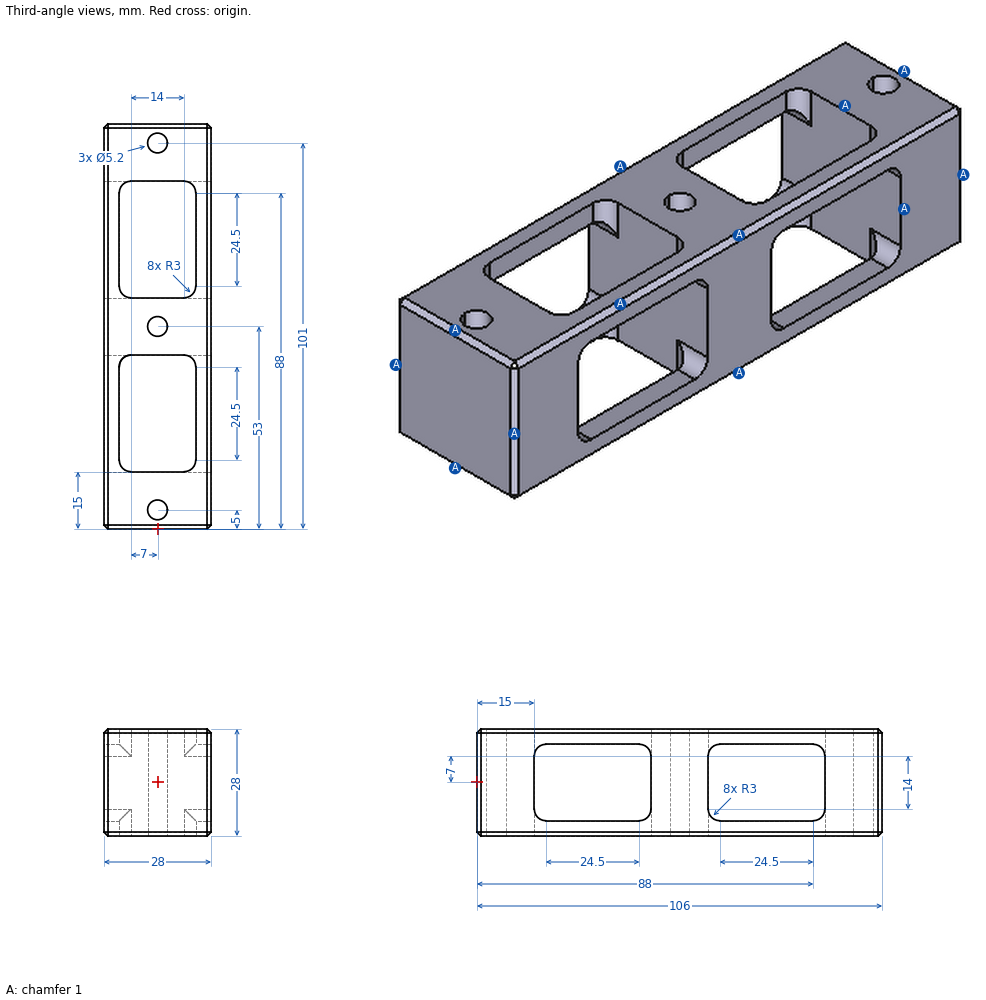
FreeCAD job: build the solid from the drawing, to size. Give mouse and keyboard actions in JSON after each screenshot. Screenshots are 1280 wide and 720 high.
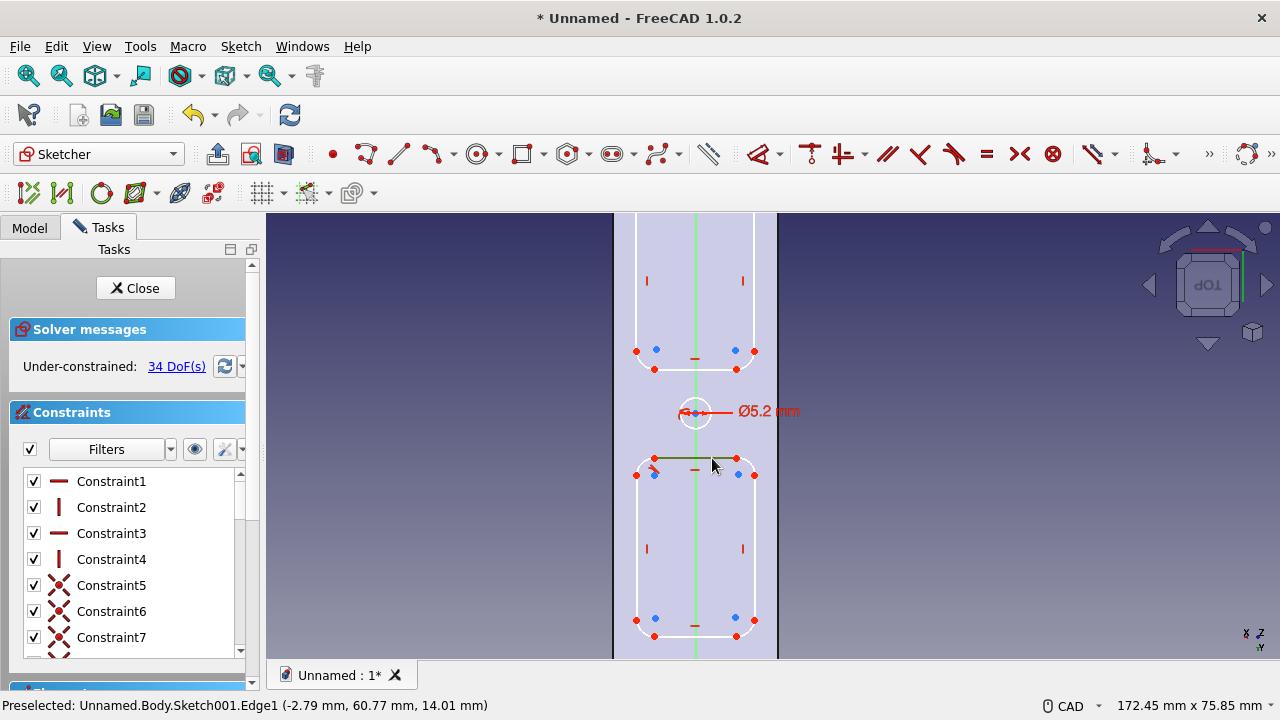
{"action": "left_click", "coordinate": [750, 463]}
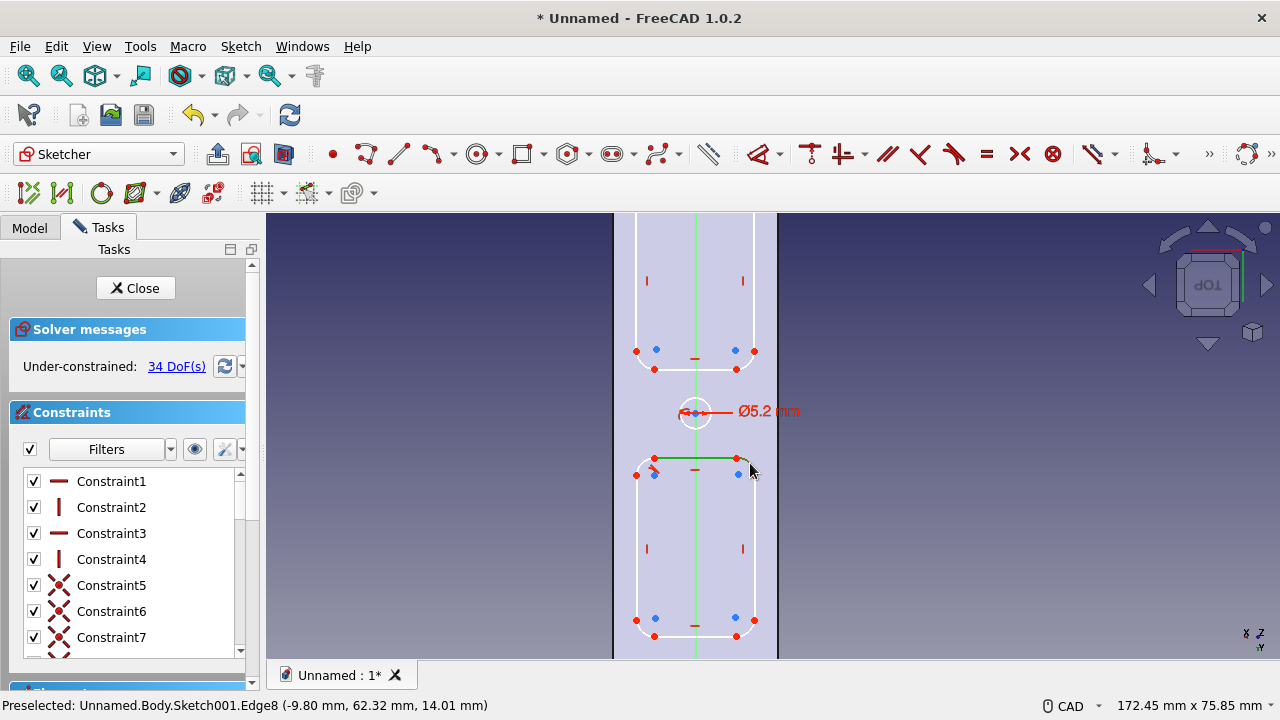
{"action": "left_click", "coordinate": [954, 154]}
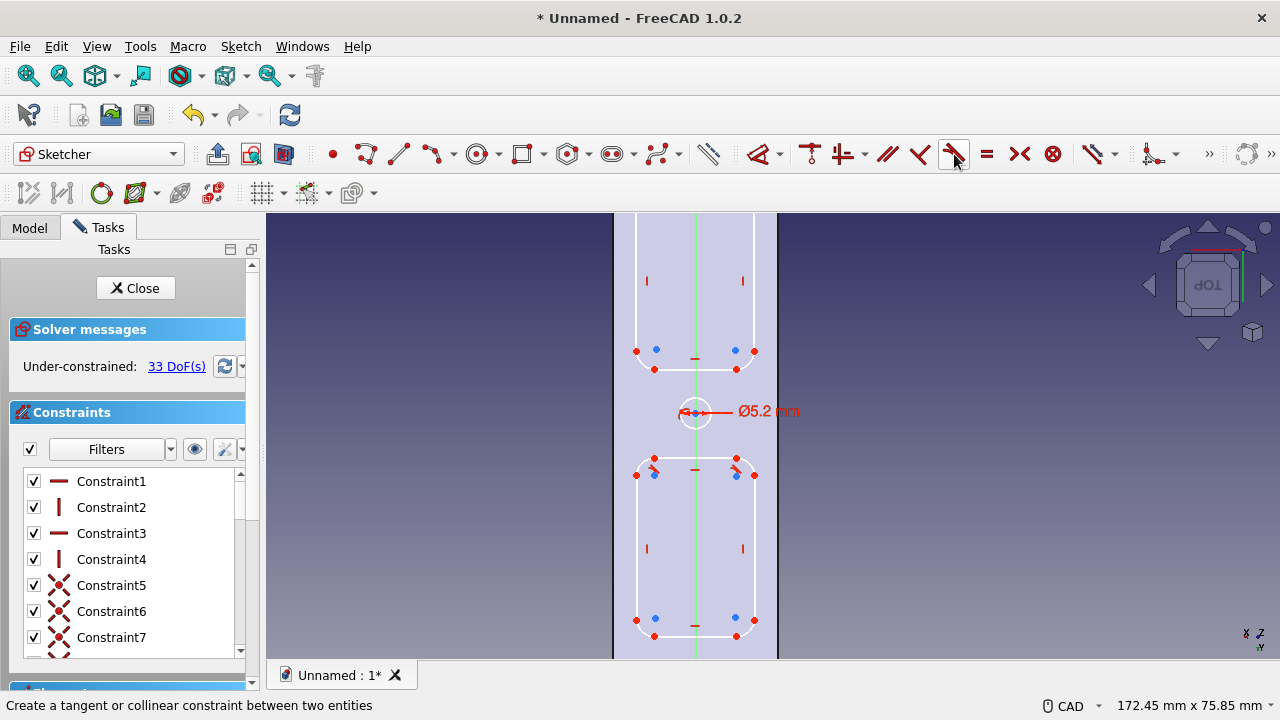
{"action": "left_click", "coordinate": [637, 519]}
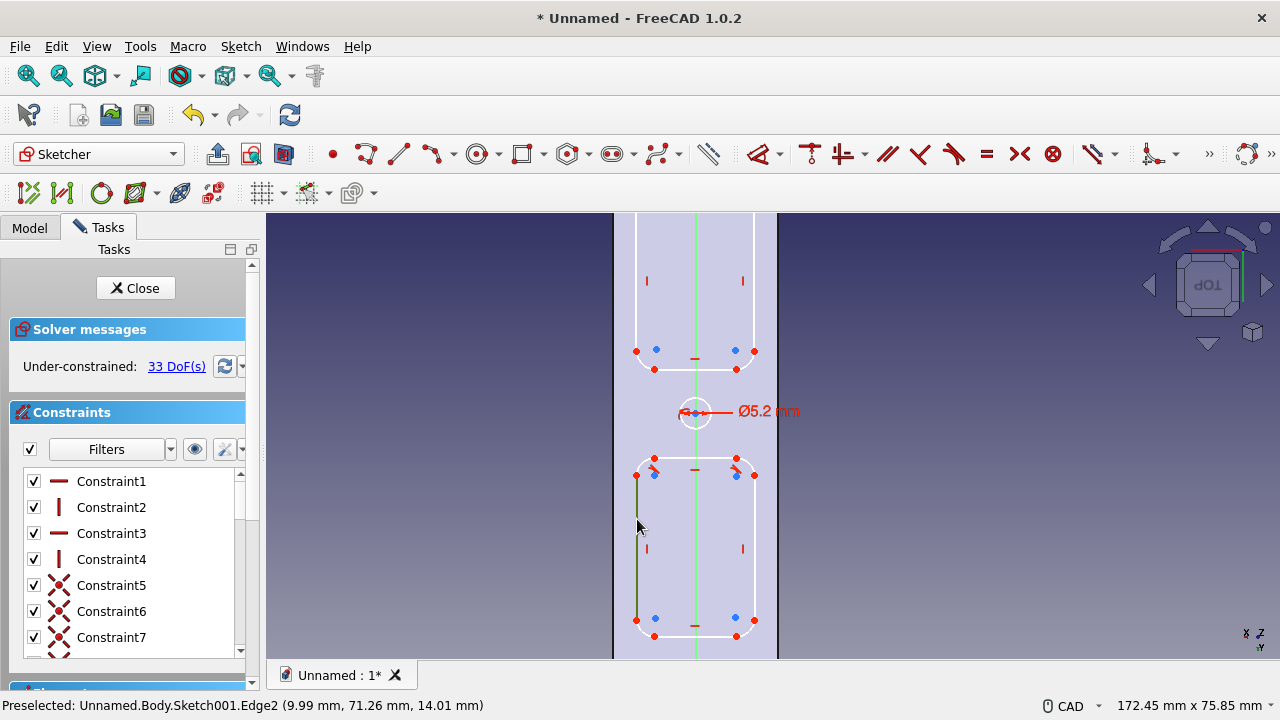
{"action": "left_click", "coordinate": [642, 463]}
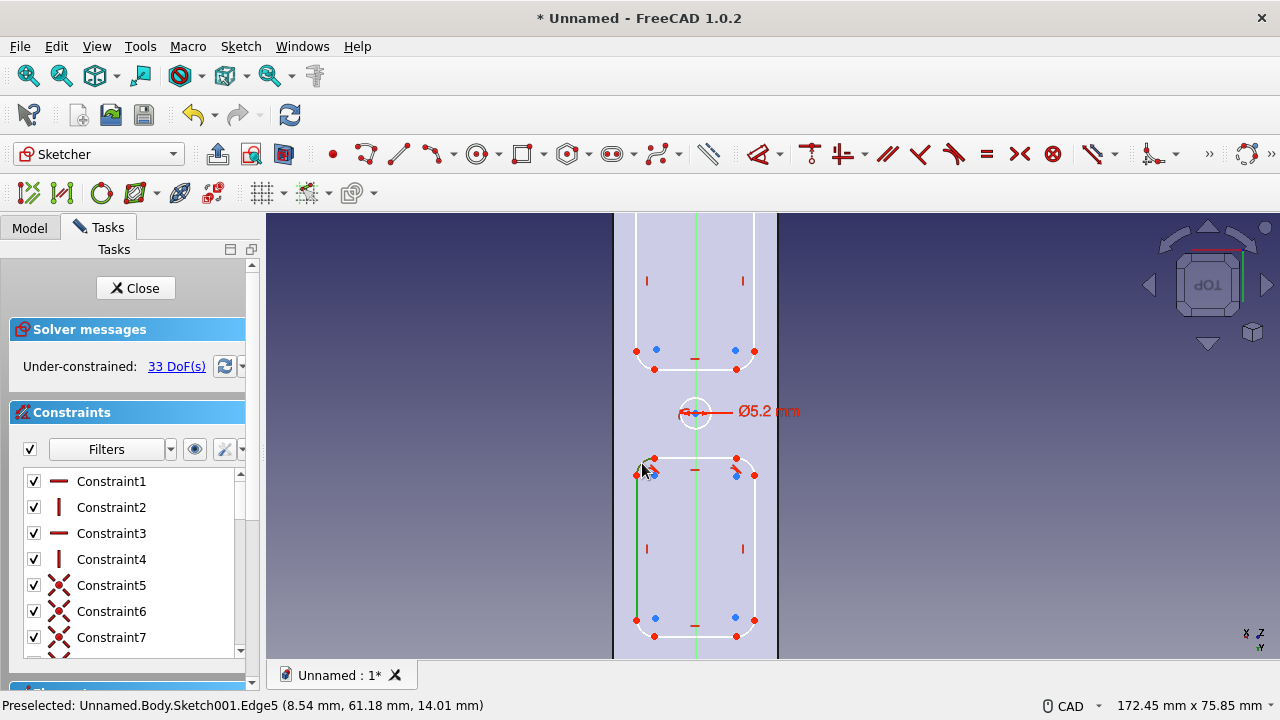
{"action": "left_click", "coordinate": [954, 154]}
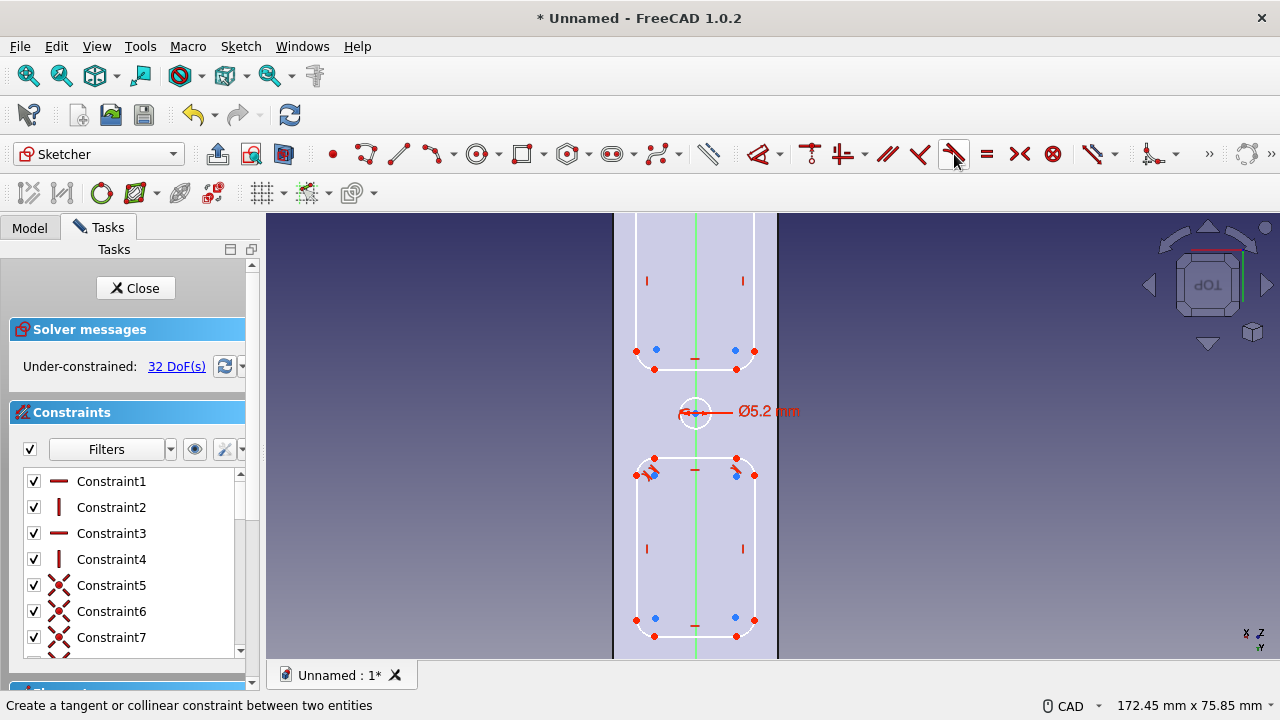
{"action": "left_click", "coordinate": [637, 519]}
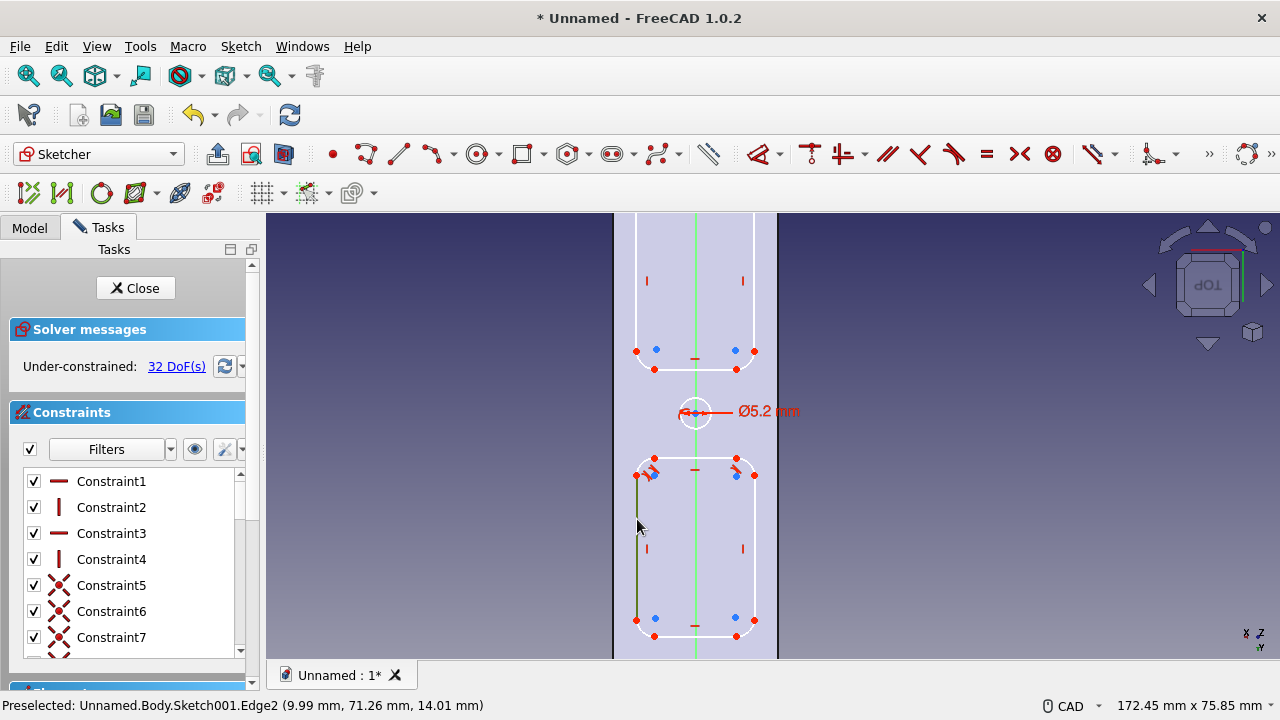
{"action": "scroll", "coordinate": [712, 461], "scroll_direction": "down", "scroll_amount": 4}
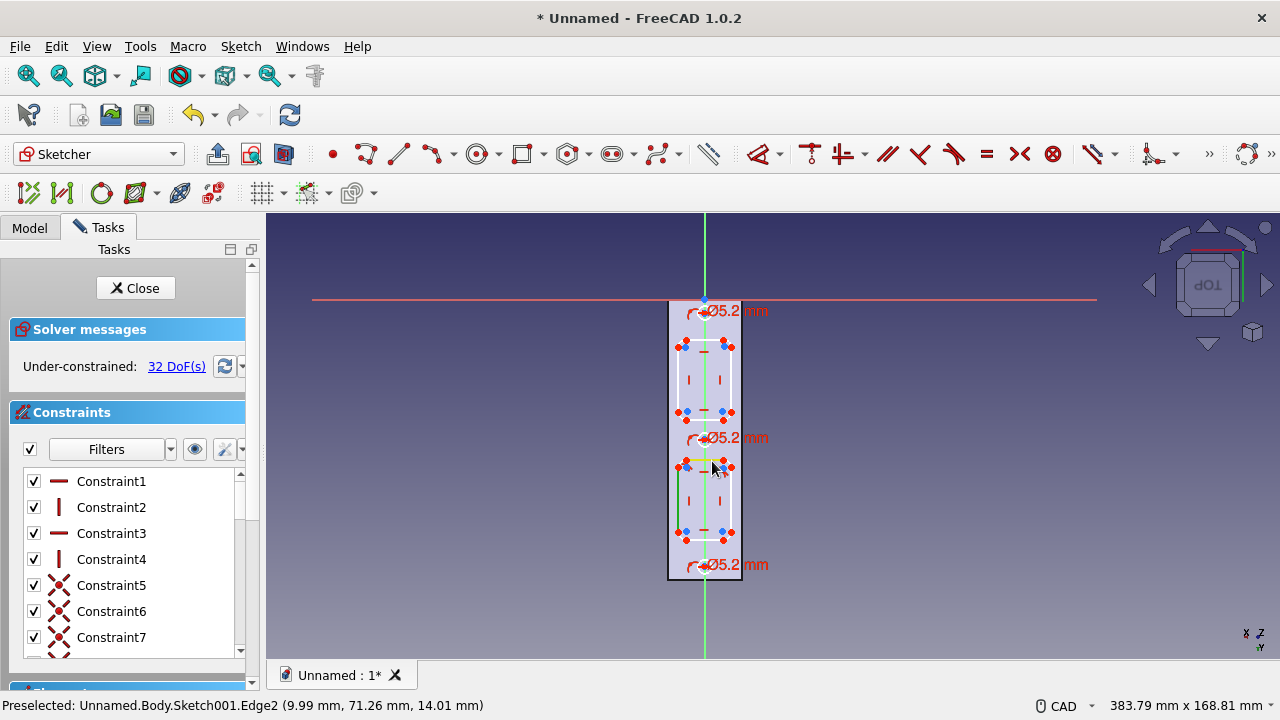
{"action": "scroll", "coordinate": [681, 538], "scroll_direction": "up", "scroll_amount": 5}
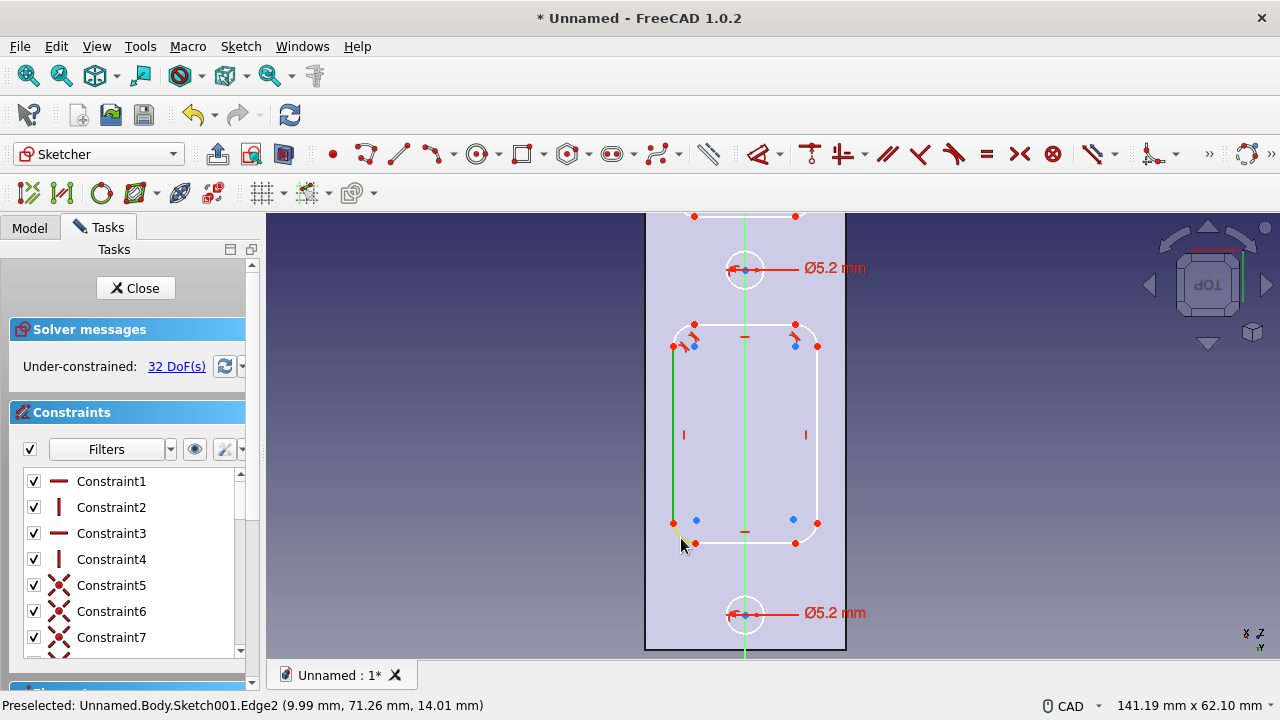
{"action": "left_click", "coordinate": [681, 537]}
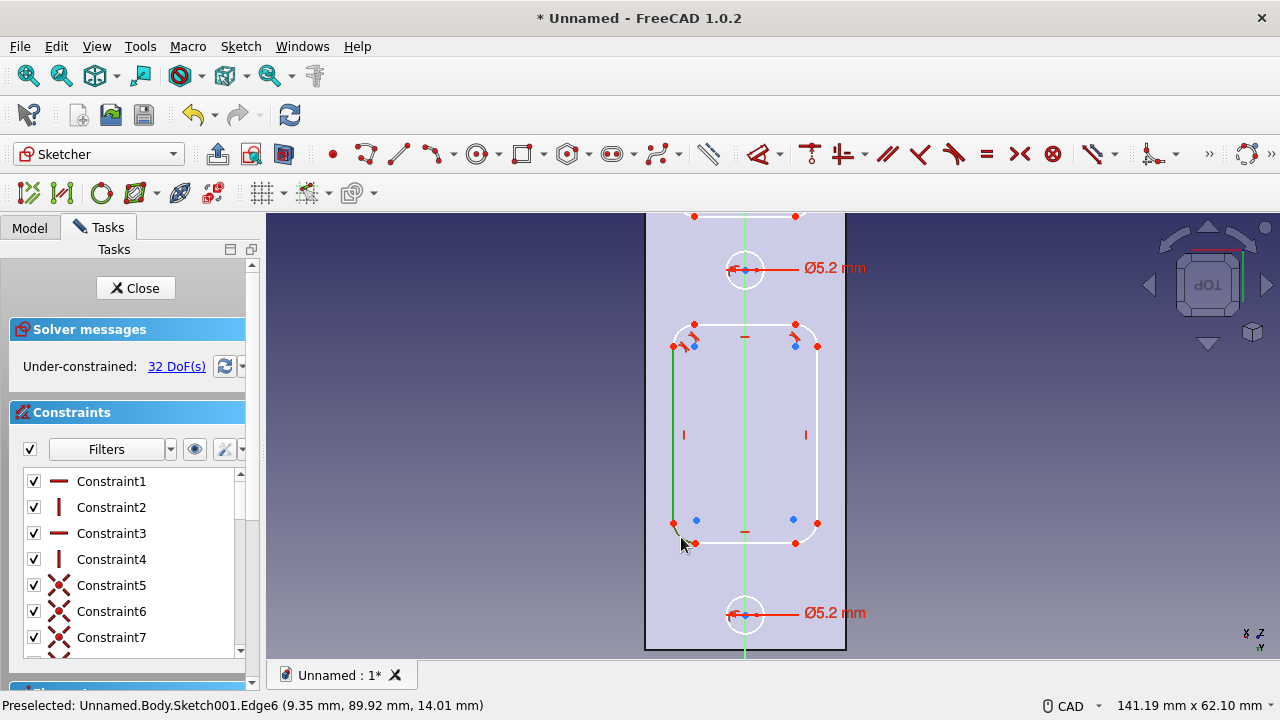
{"action": "left_click", "coordinate": [954, 154]}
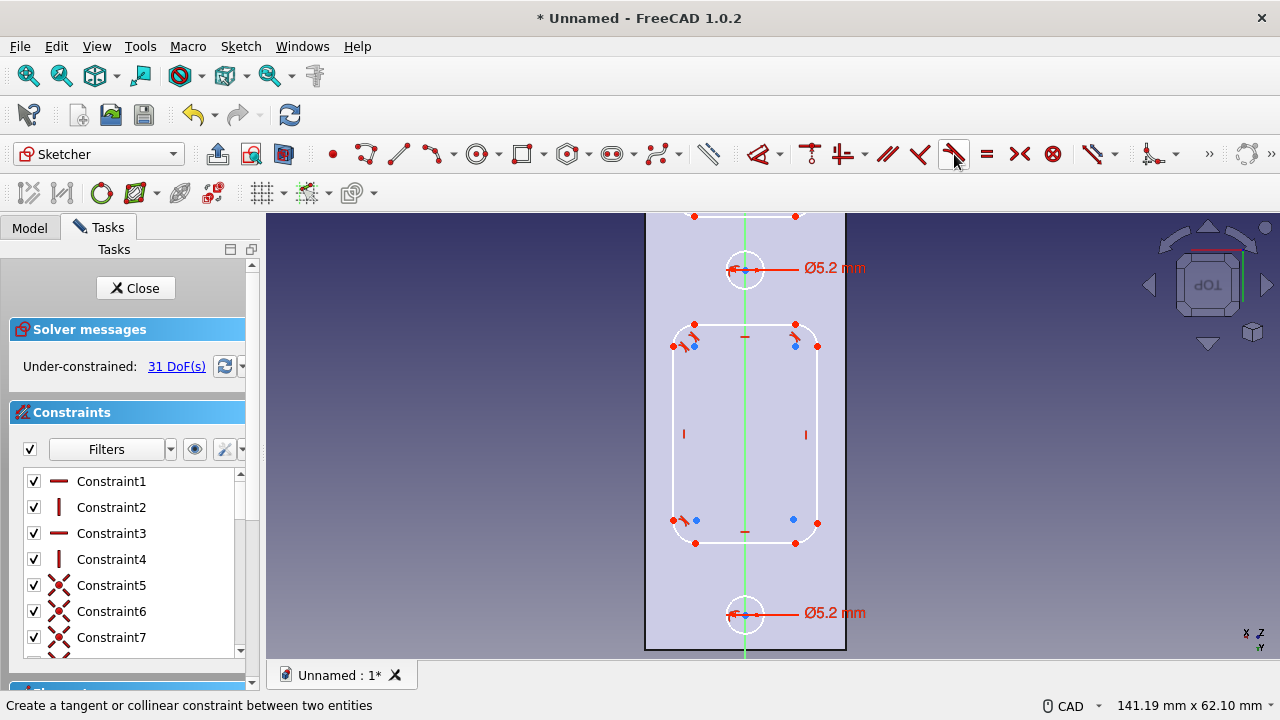
{"action": "left_click", "coordinate": [725, 543]}